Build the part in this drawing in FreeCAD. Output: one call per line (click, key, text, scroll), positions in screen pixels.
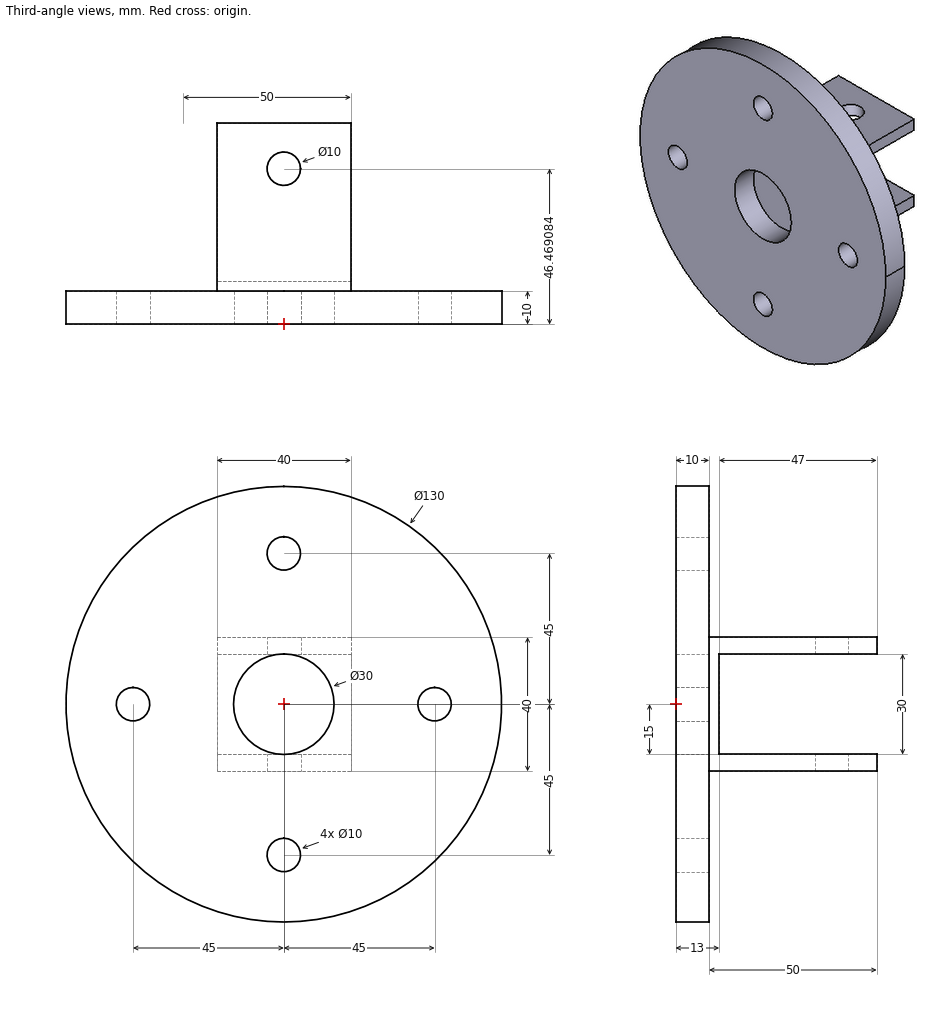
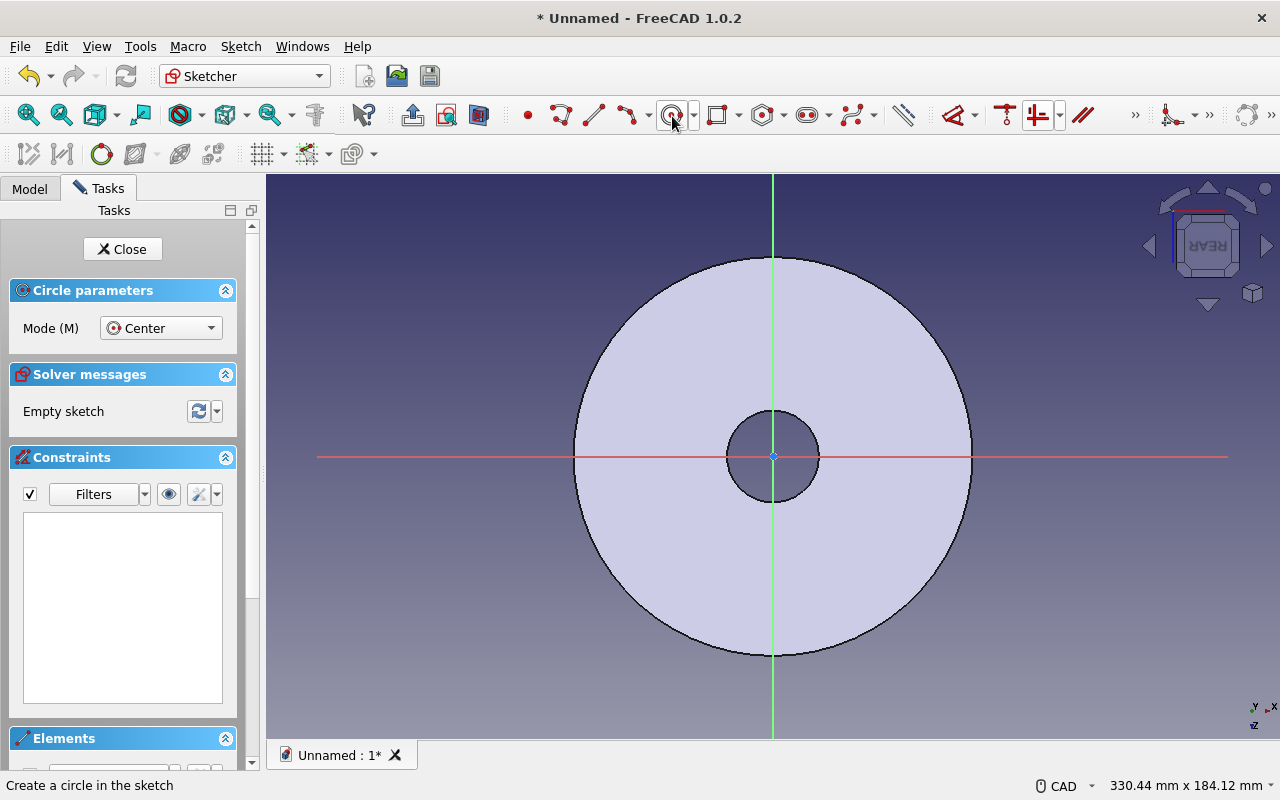
scroll(773, 318, up, 2)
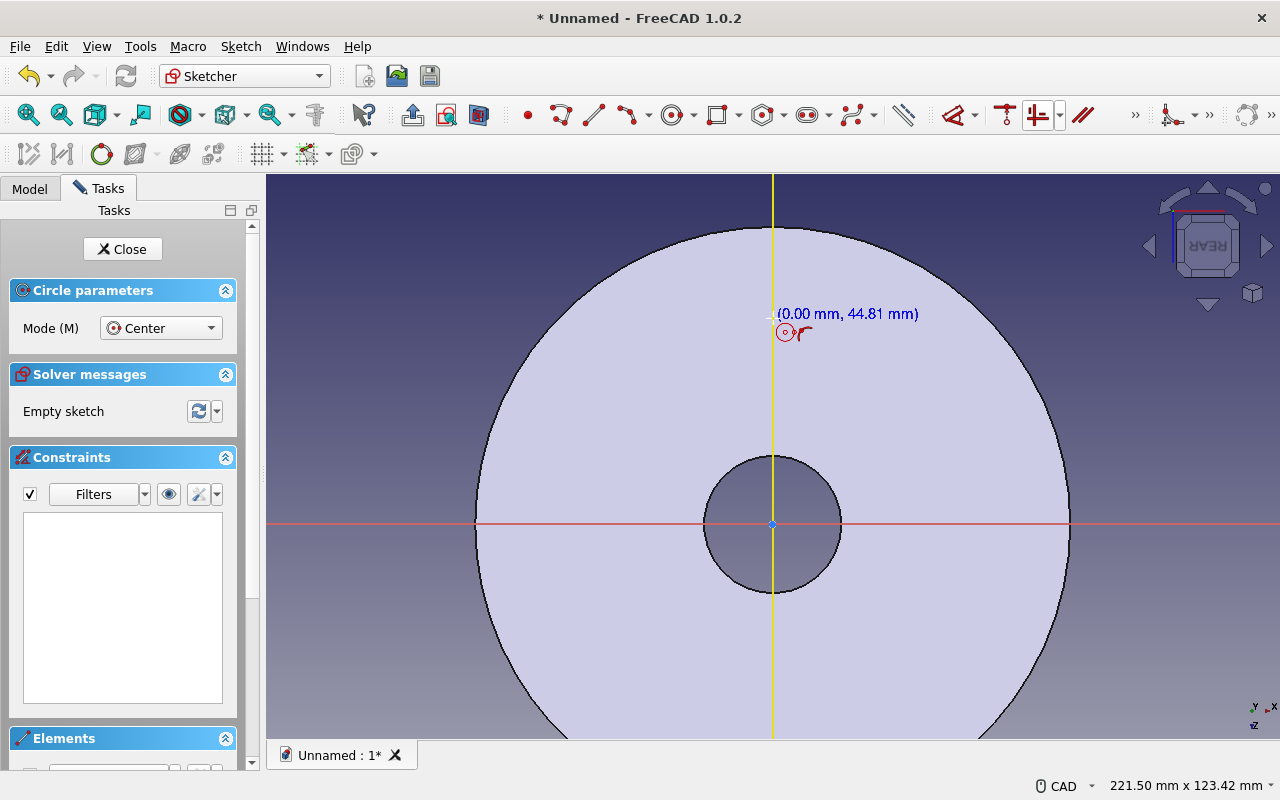
click(773, 318)
move(789, 302)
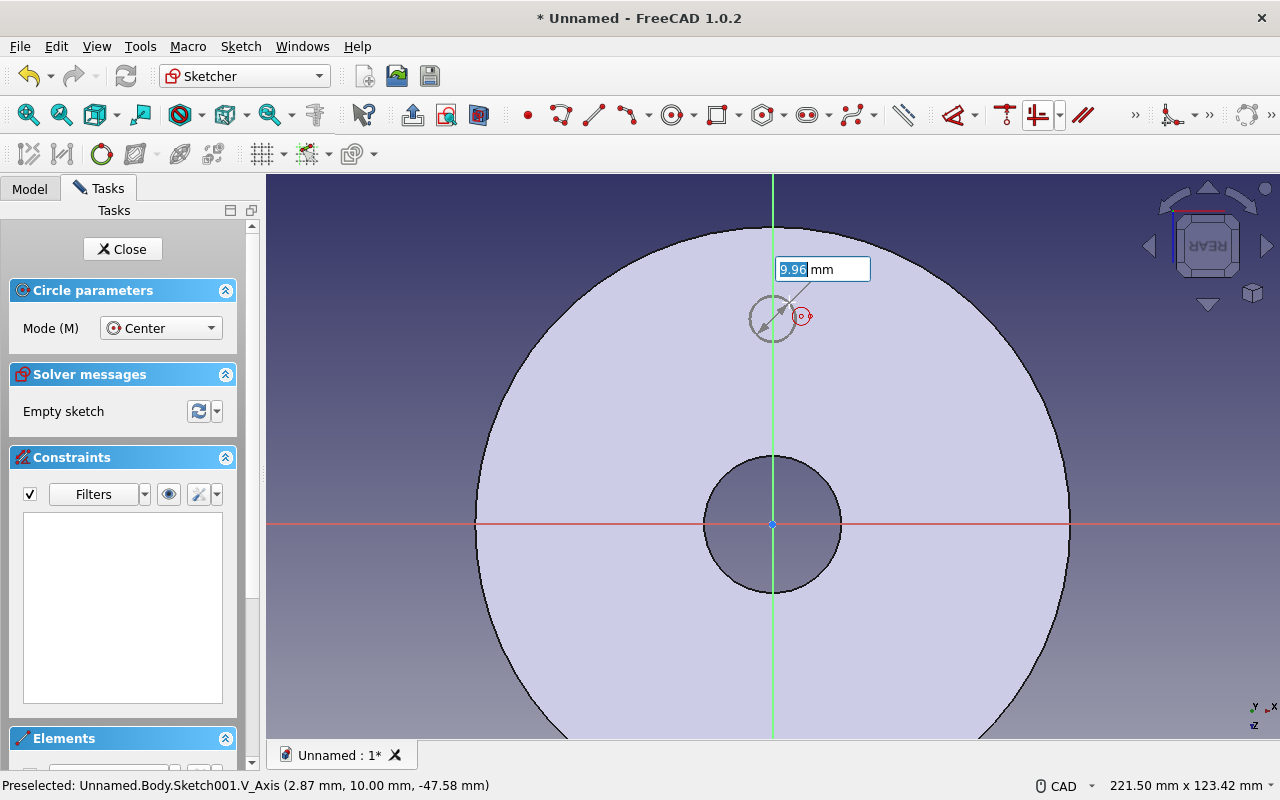
text(10)
key(Return)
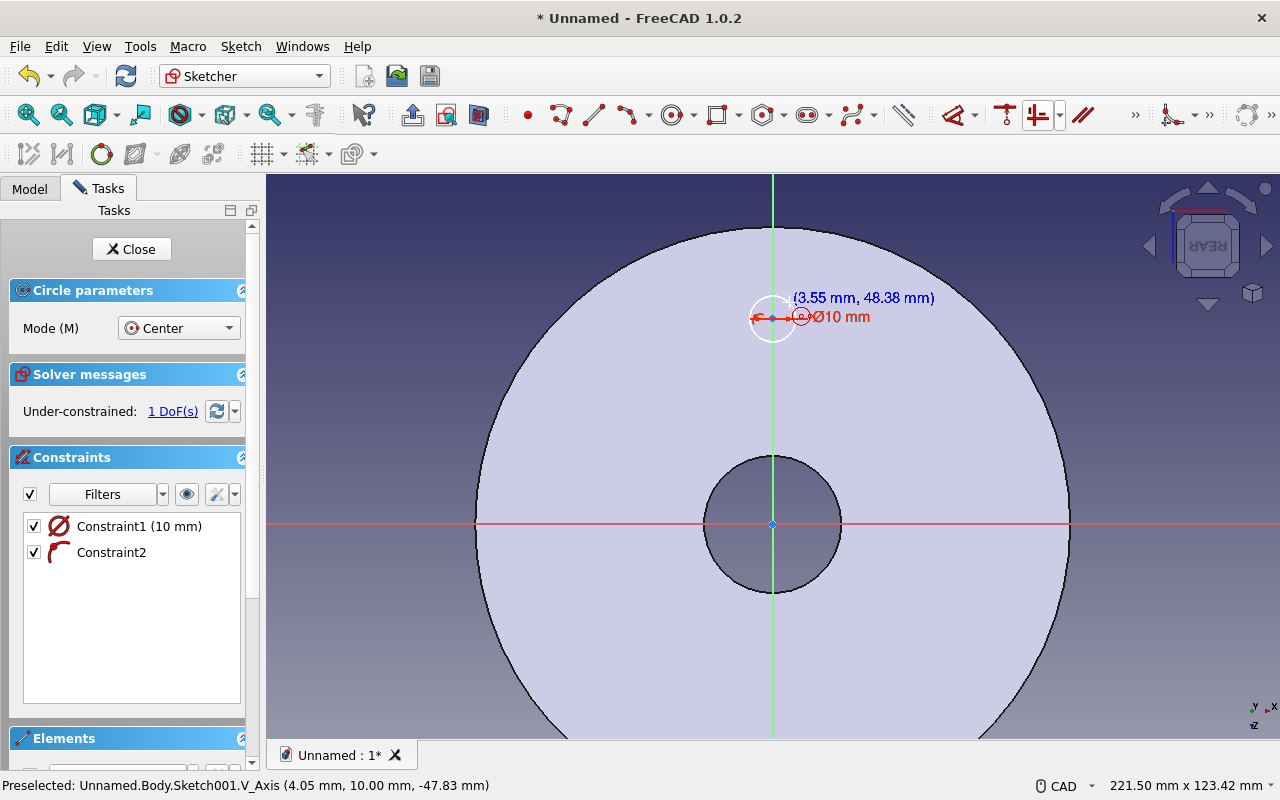
click(979, 524)
move(995, 508)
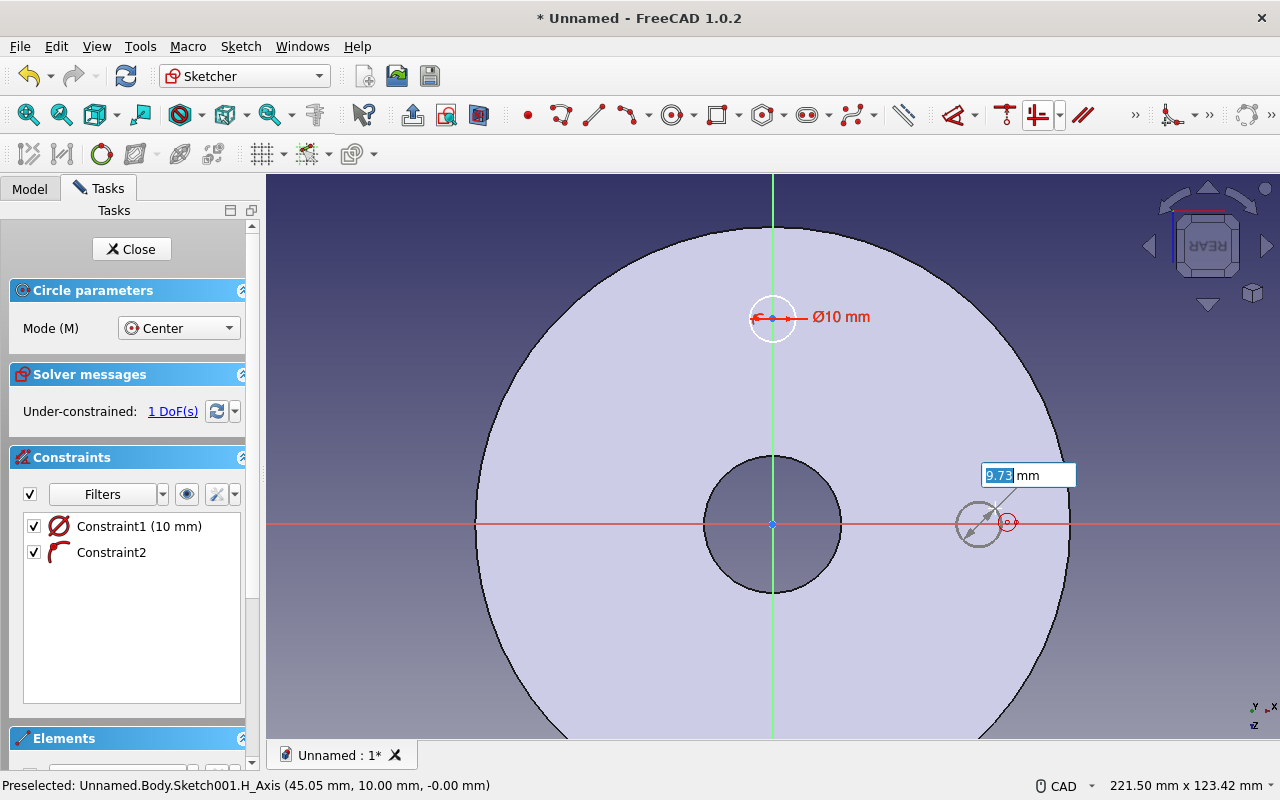
text(10)
key(Return)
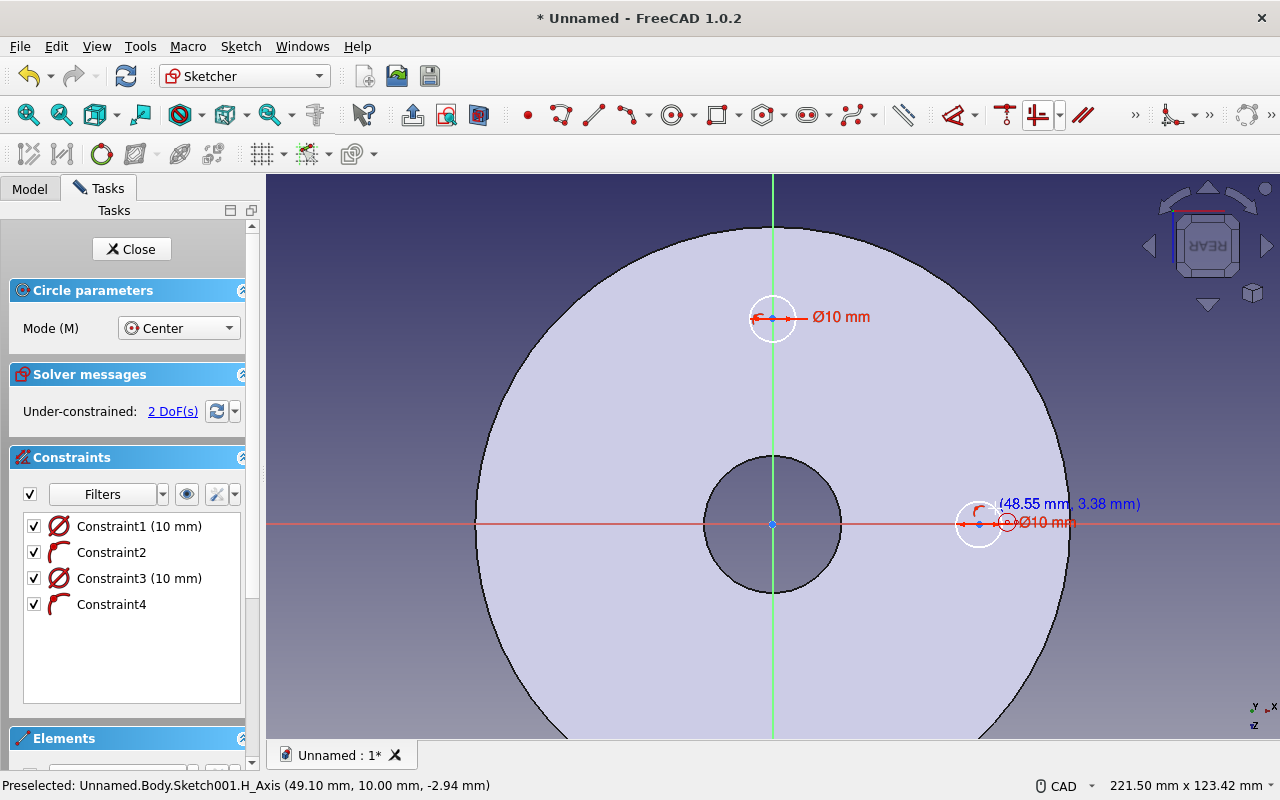
scroll(396, 202, down, 1)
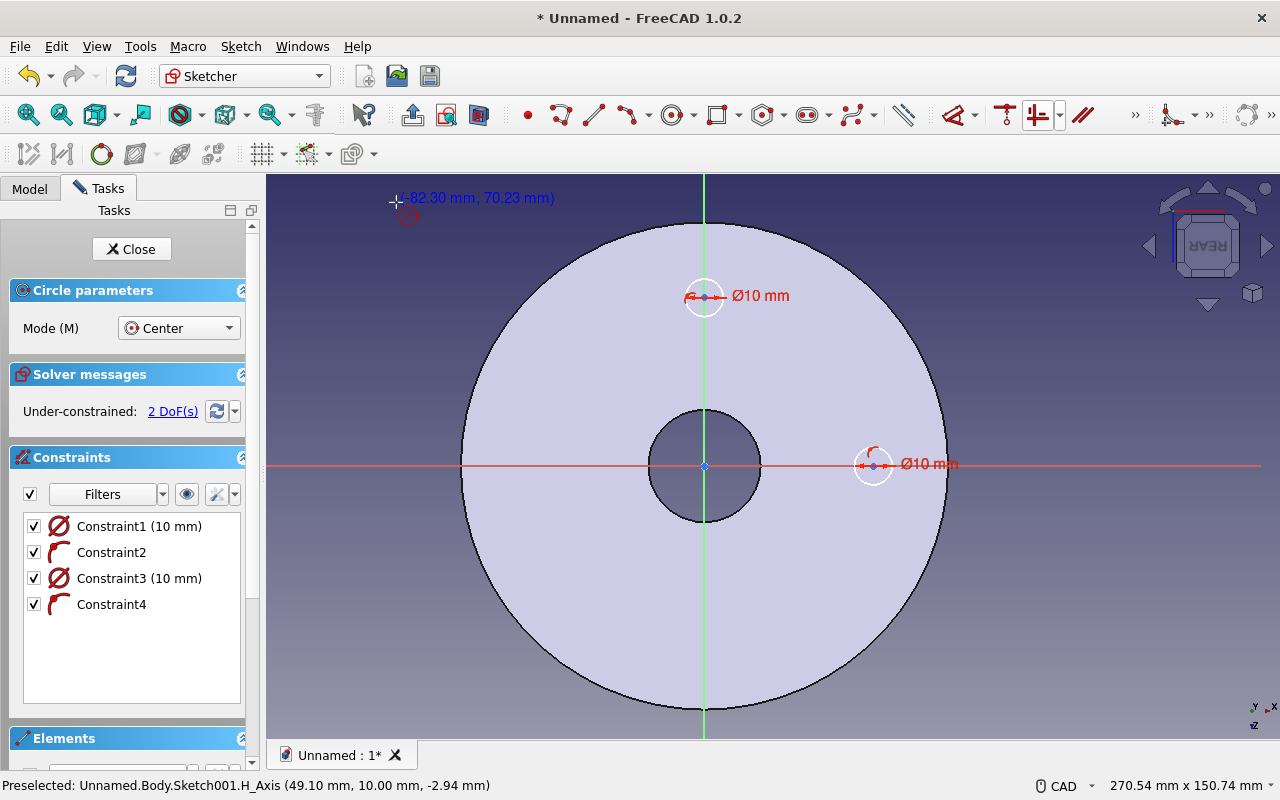
click(704, 635)
move(722, 628)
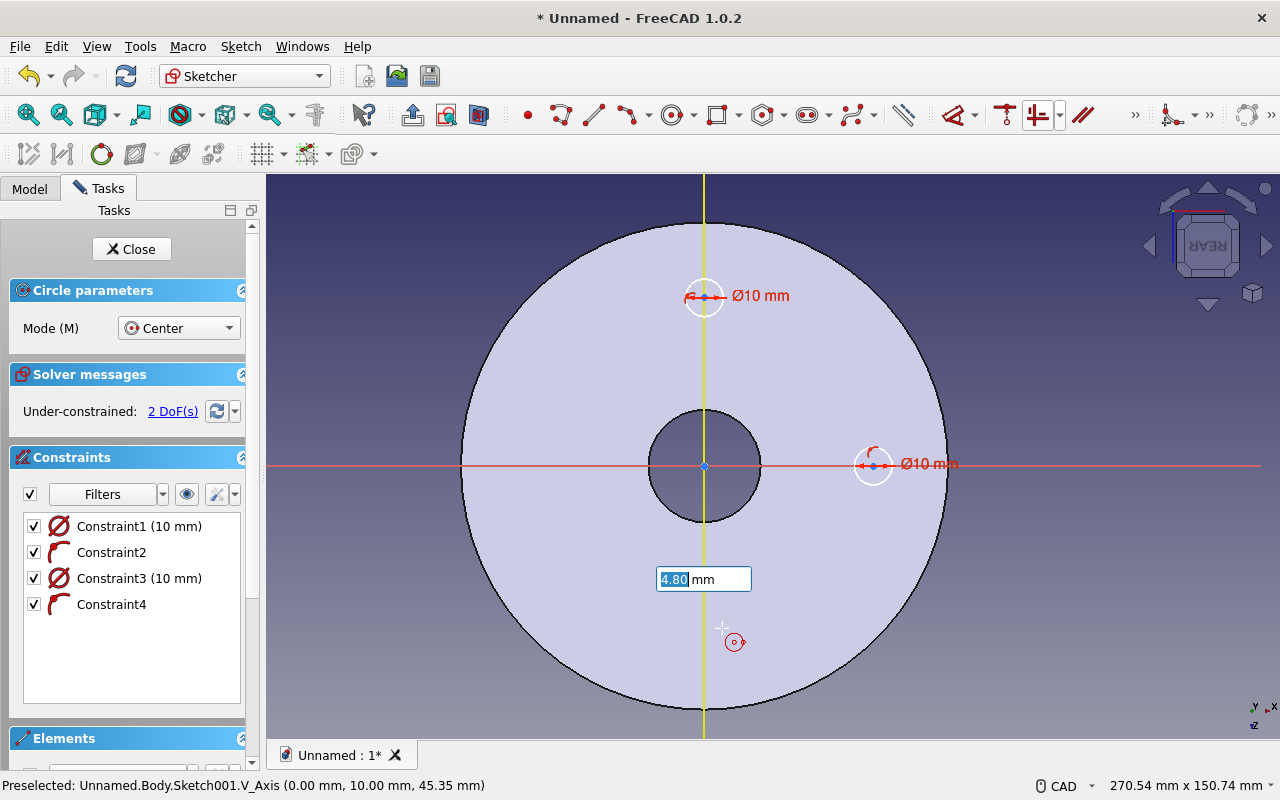
text(10)
key(Return)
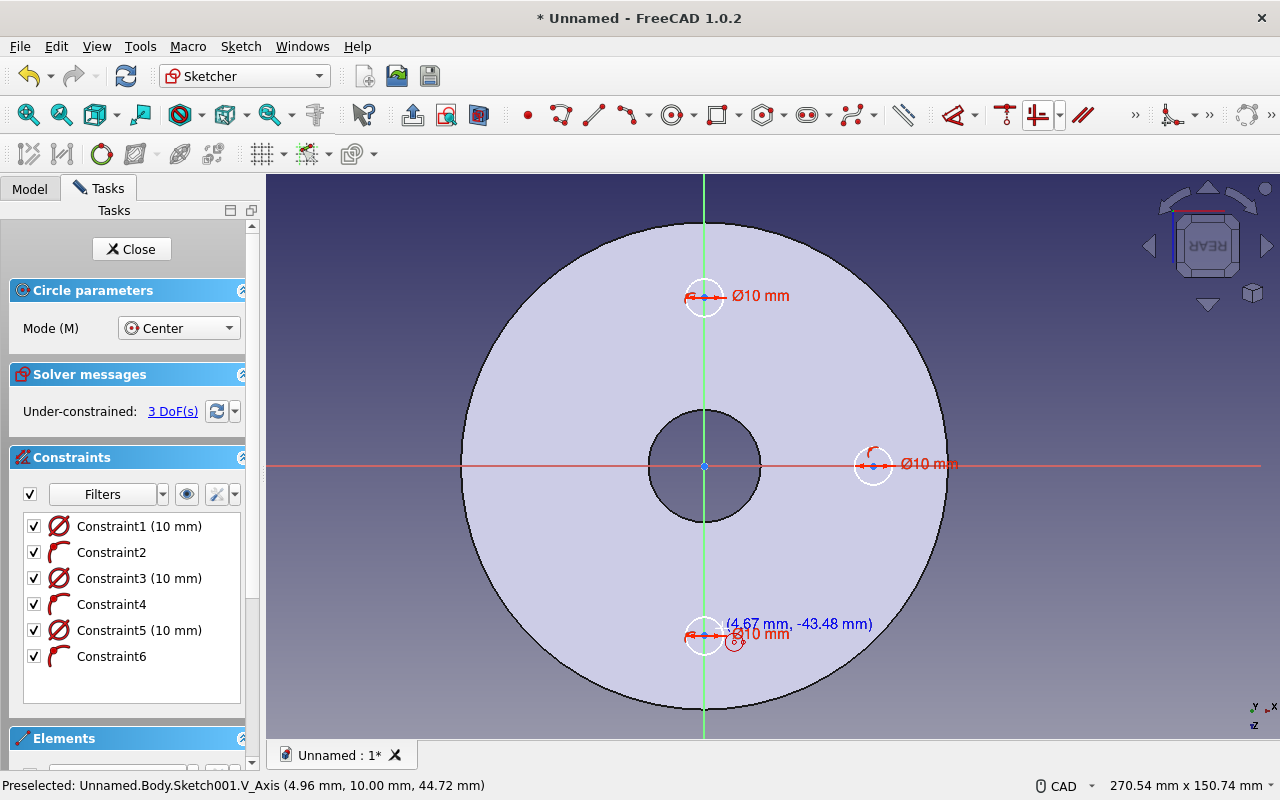
click(536, 466)
move(542, 448)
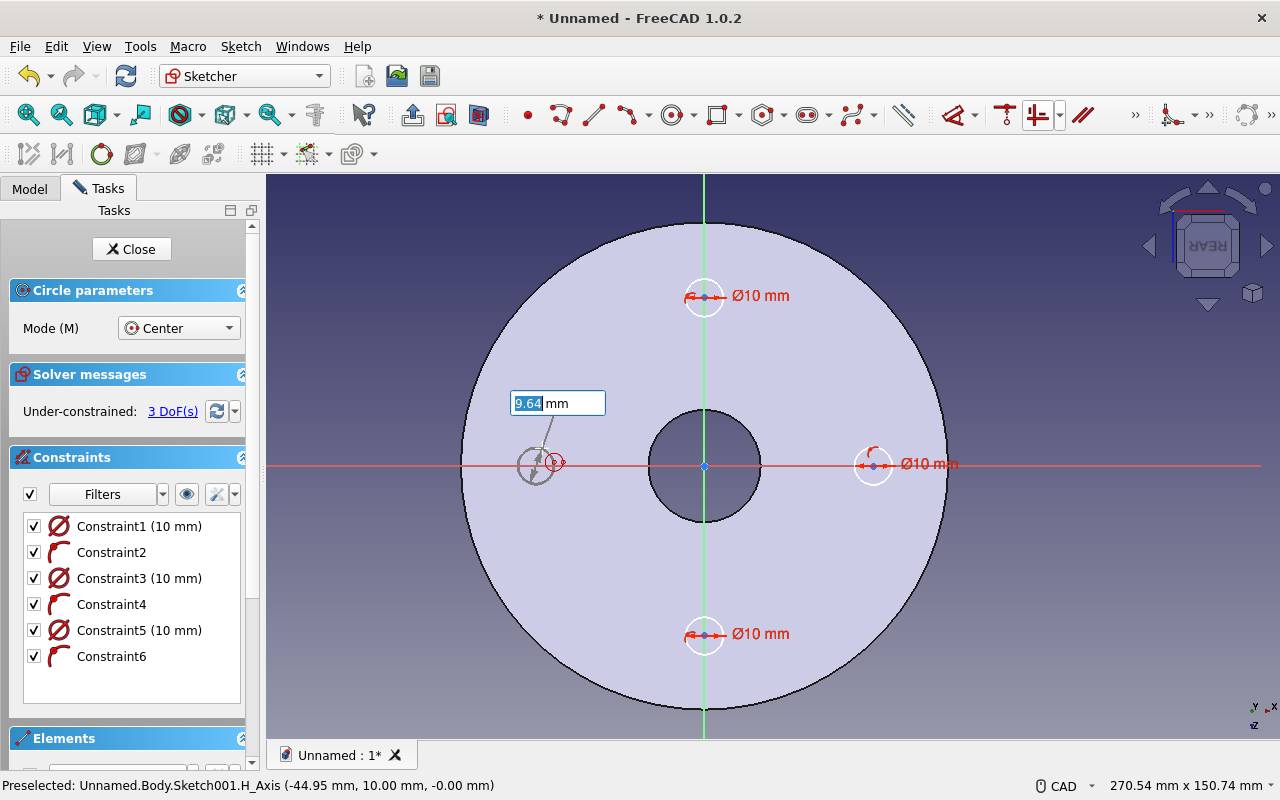
text(10)
key(Return)
key(Escape)